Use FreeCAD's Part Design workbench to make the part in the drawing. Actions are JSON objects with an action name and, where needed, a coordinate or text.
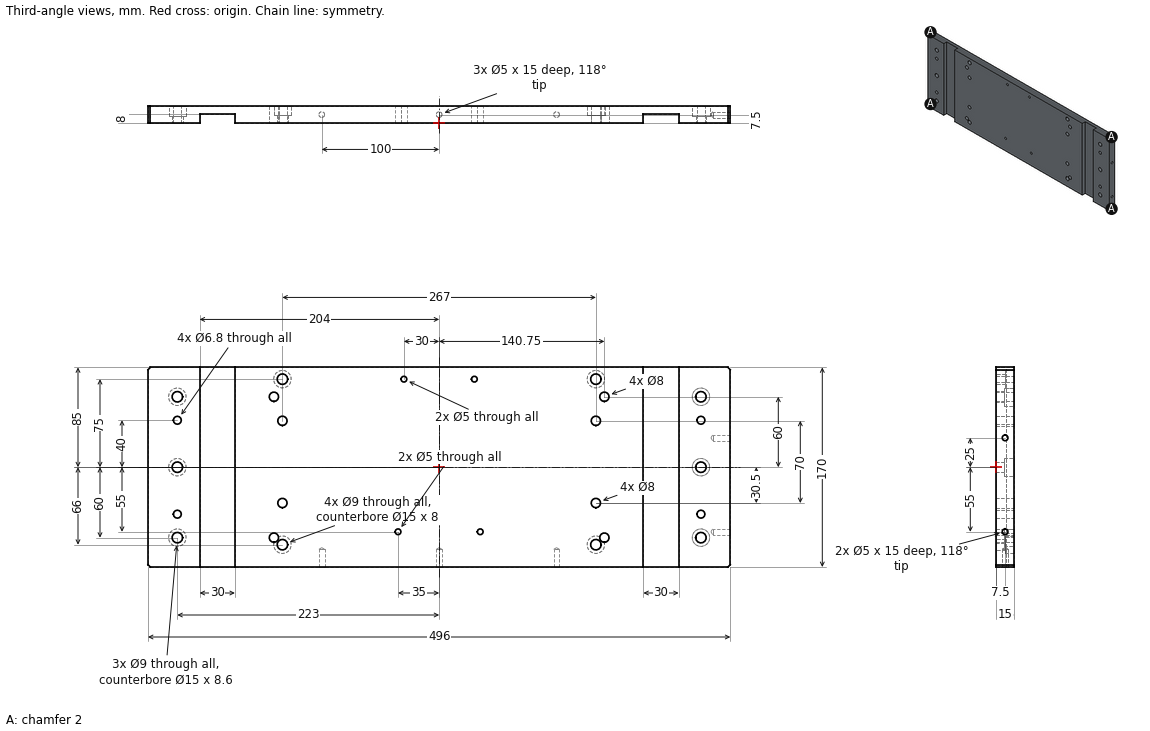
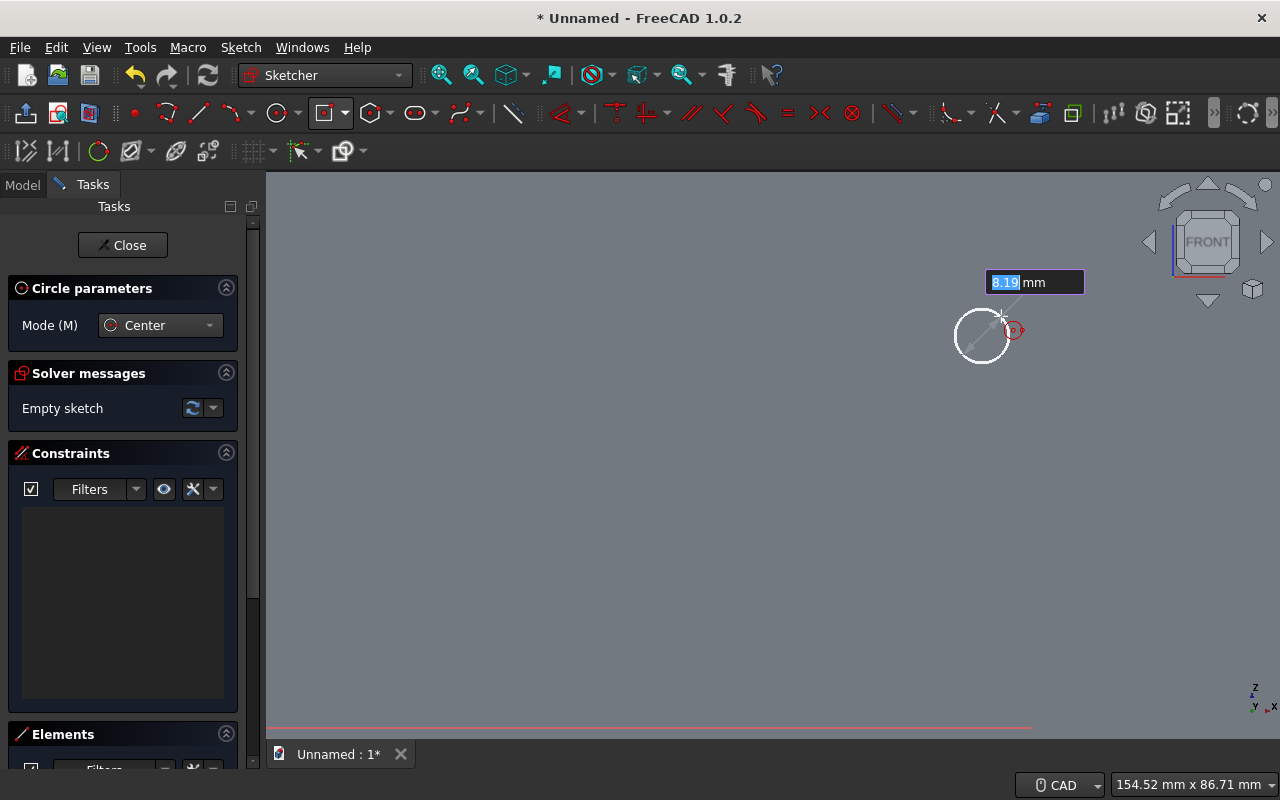
{"action": "type", "text": "8"}
{"action": "key", "text": "Return"}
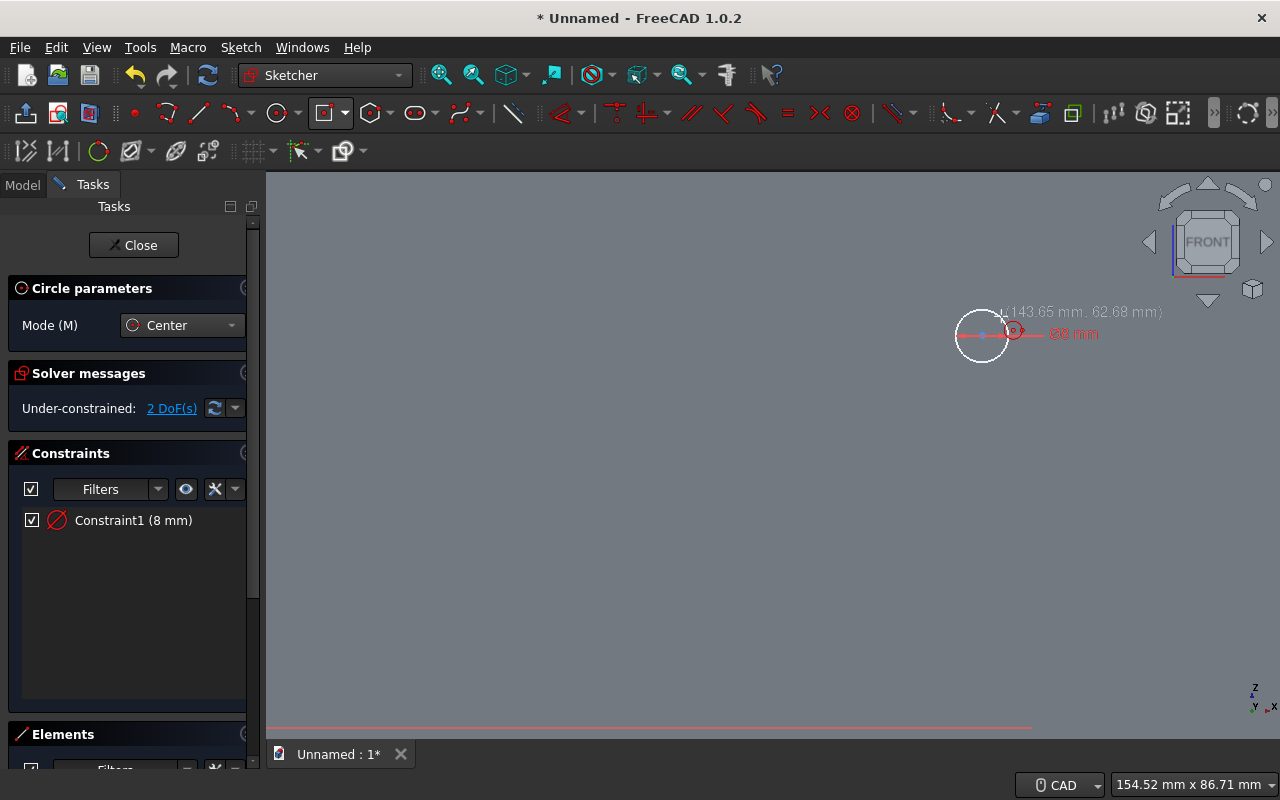
{"action": "scroll", "coordinate": [983, 336], "scroll_direction": "down", "scroll_amount": 6}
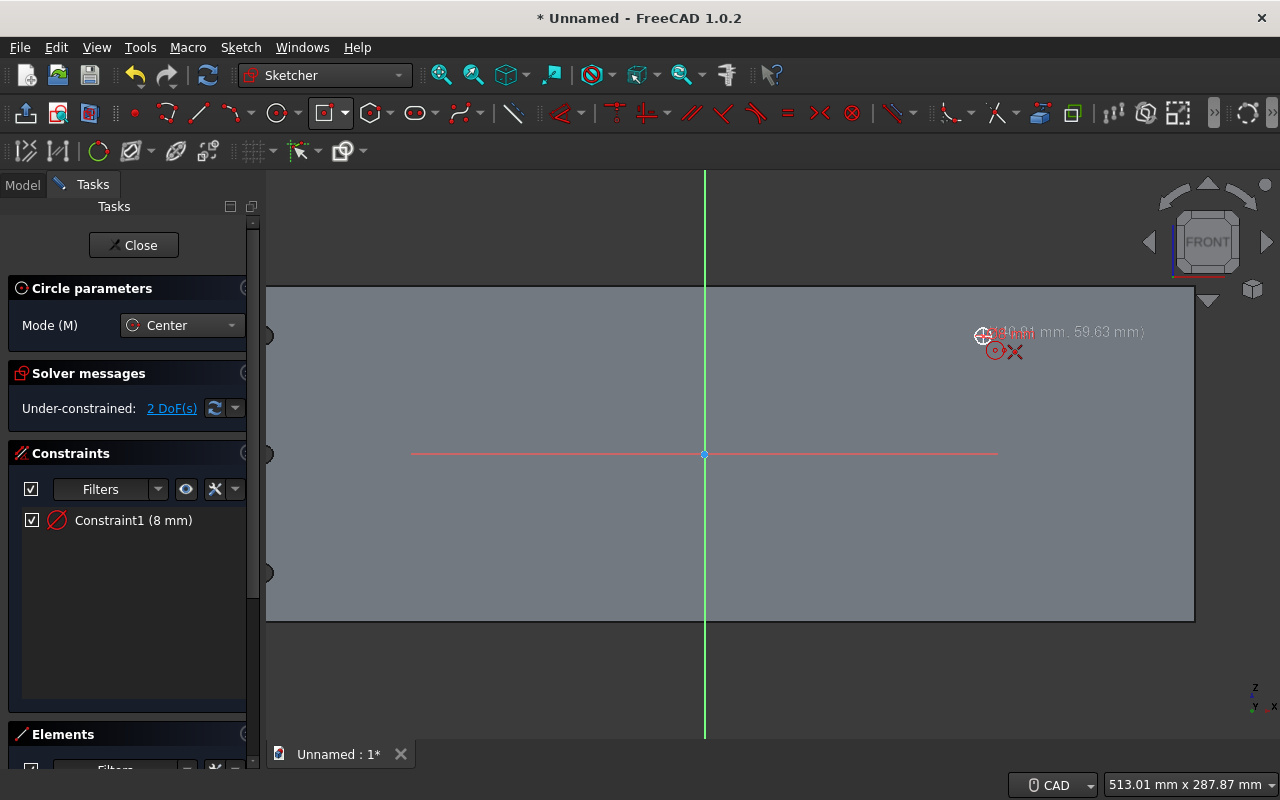
{"action": "scroll", "coordinate": [983, 573], "scroll_direction": "up", "scroll_amount": 6}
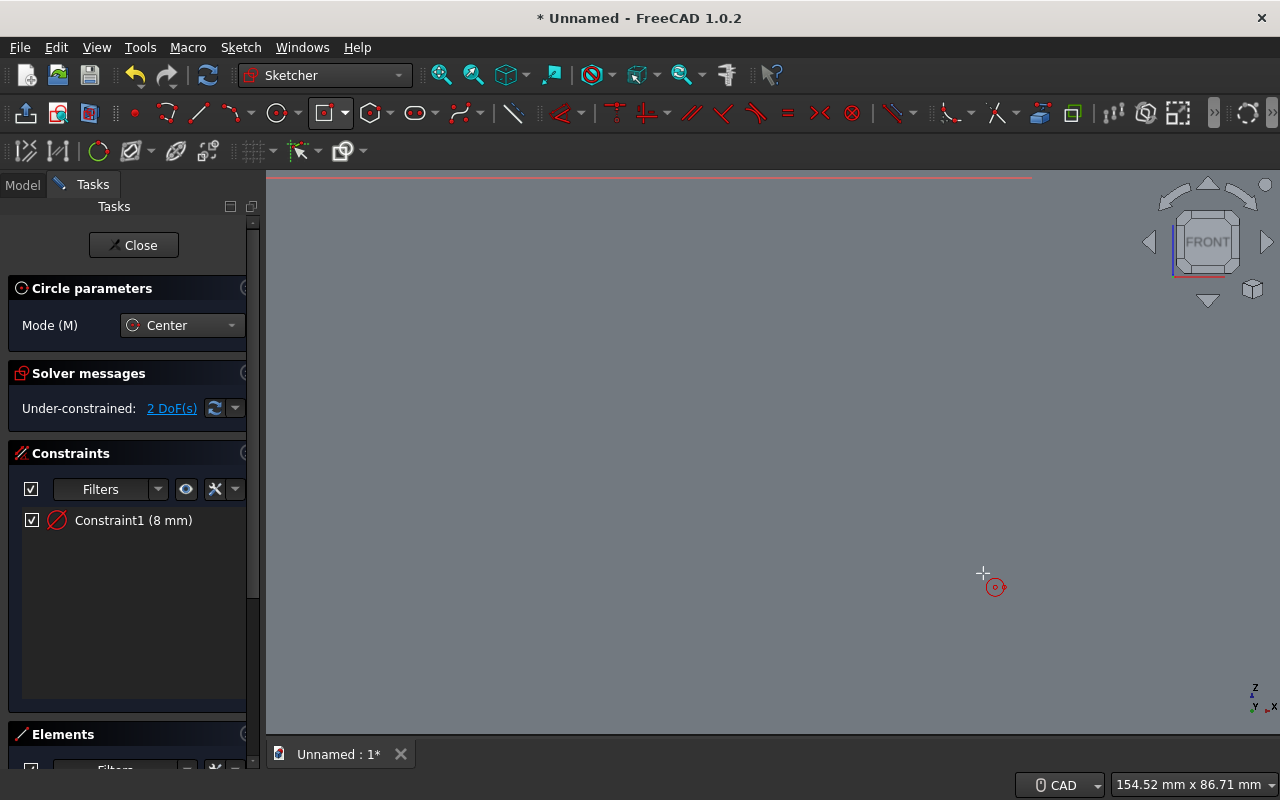
{"action": "left_click", "coordinate": [982, 571]}
{"action": "mouse_move", "coordinate": [1001, 553]}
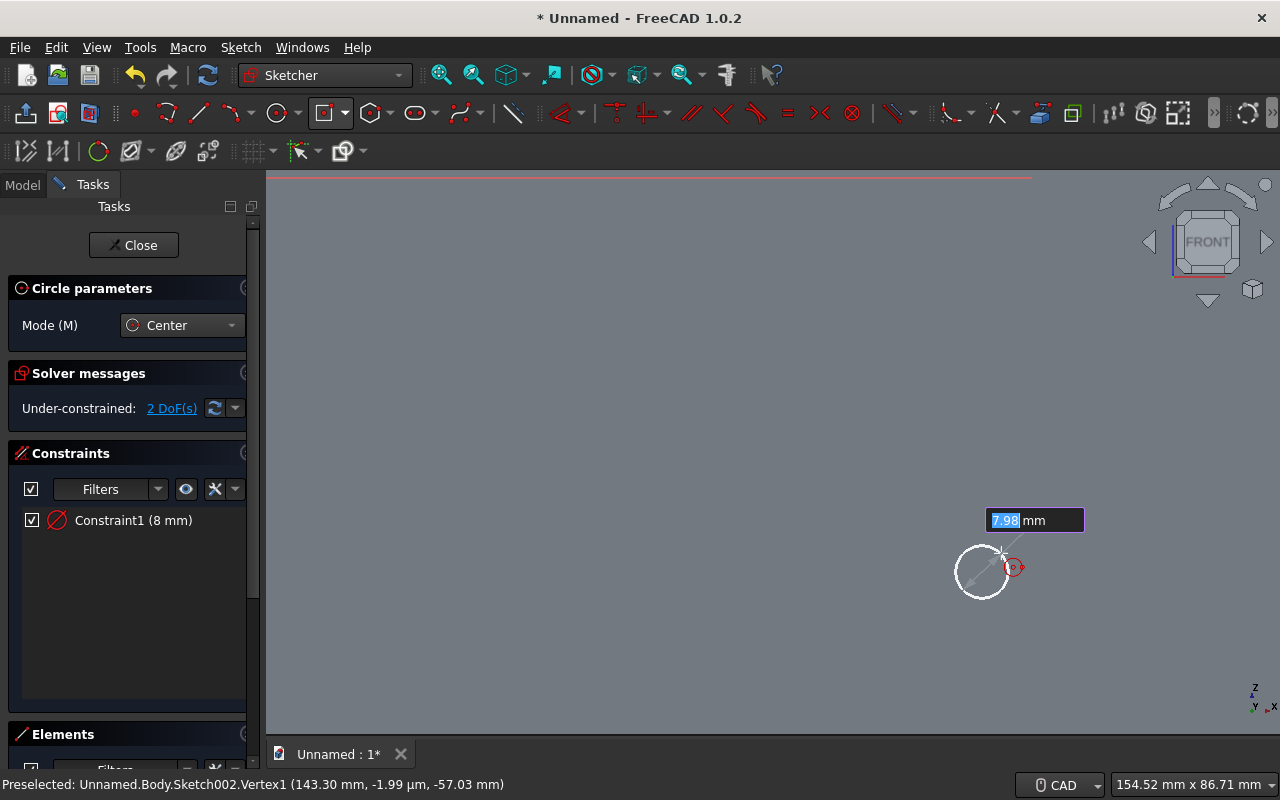
{"action": "type", "text": "8"}
{"action": "key", "text": "Return"}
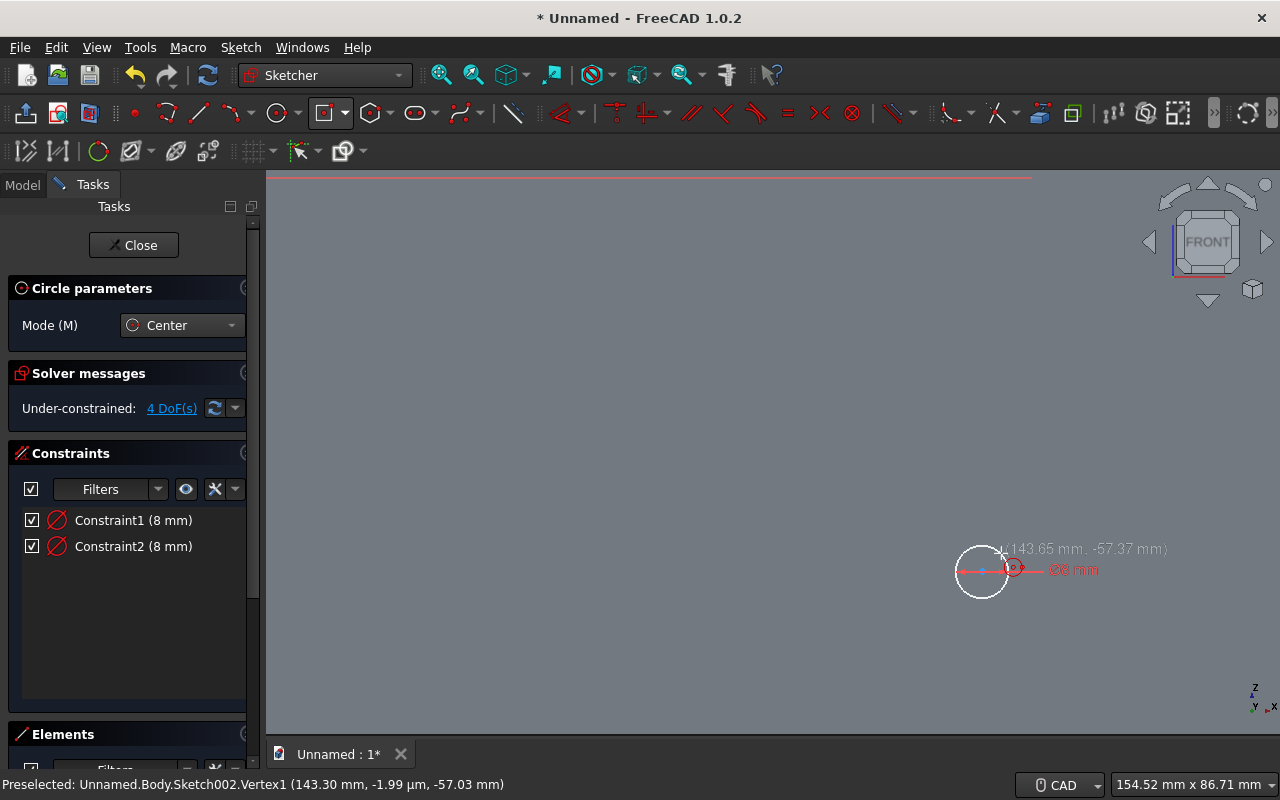
{"action": "scroll", "coordinate": [983, 574], "scroll_direction": "down", "scroll_amount": 6}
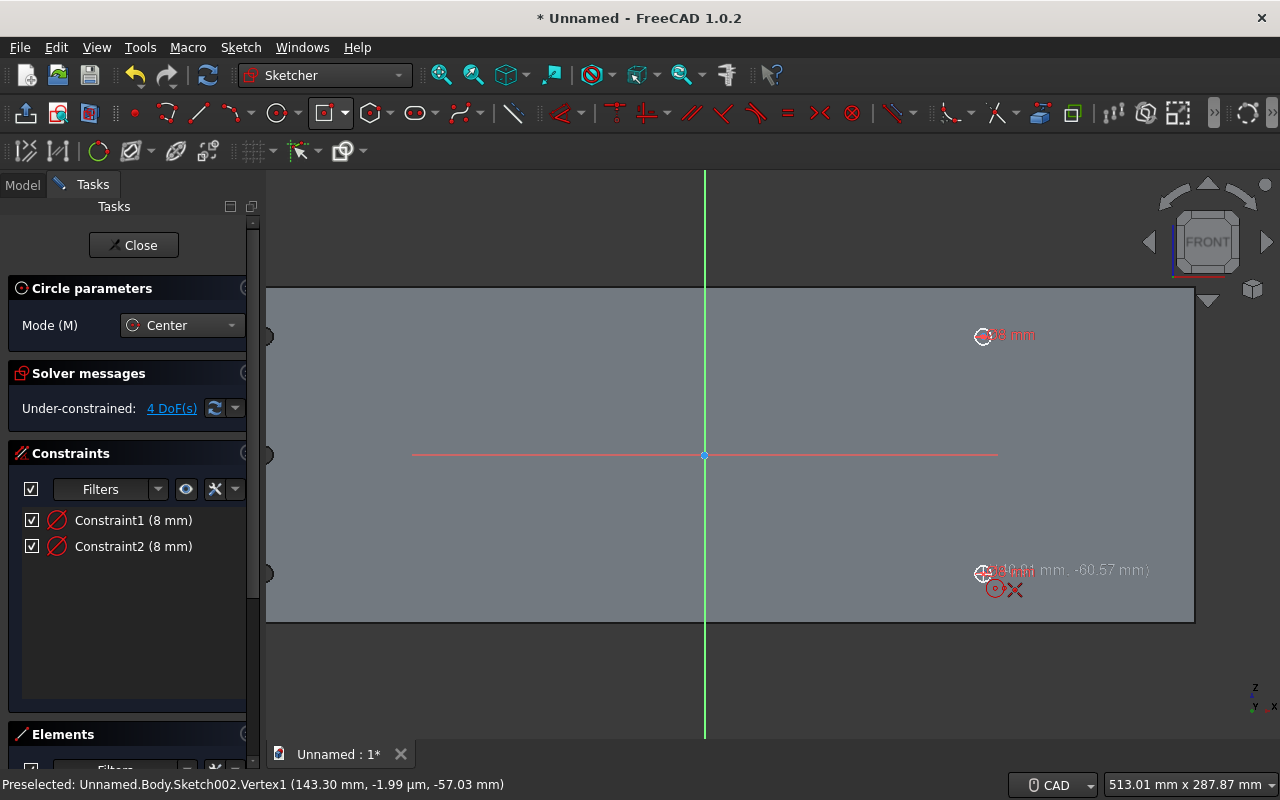
{"action": "scroll", "coordinate": [427, 574], "scroll_direction": "up", "scroll_amount": 6}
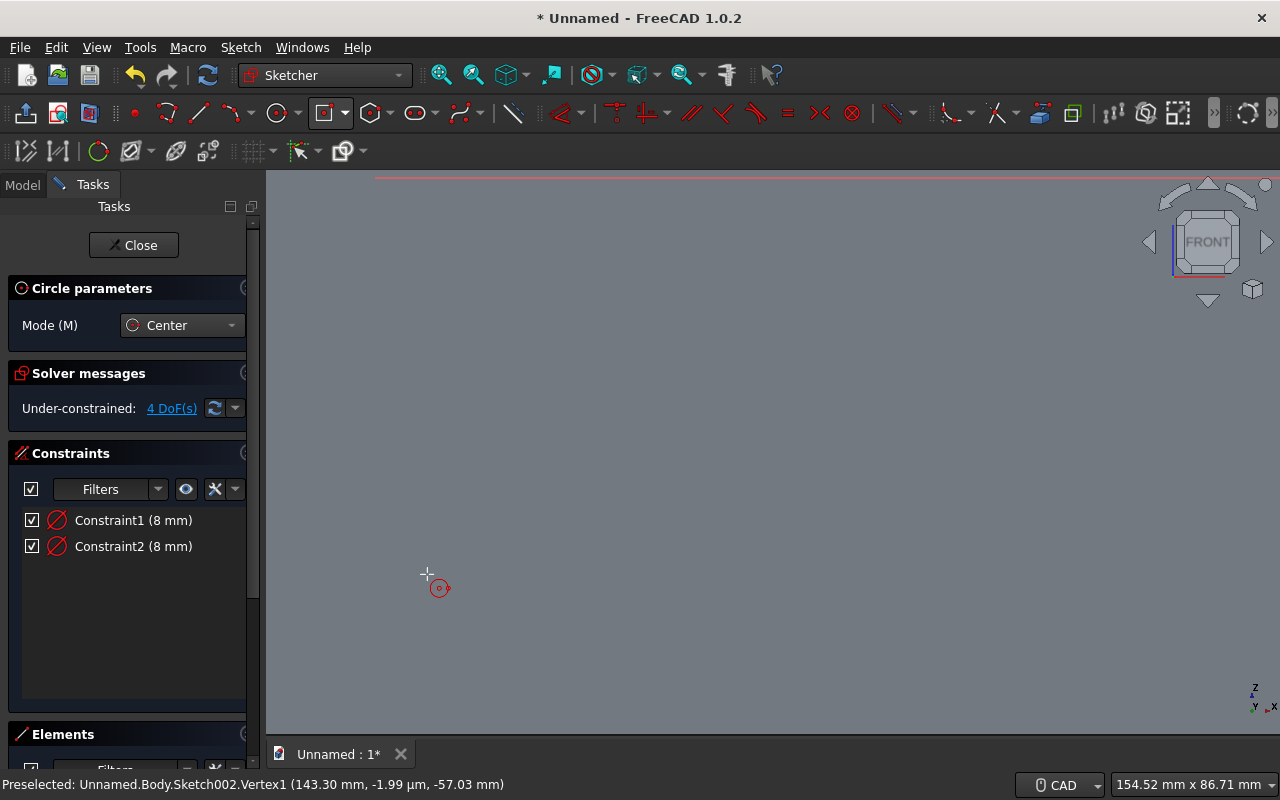
{"action": "left_click", "coordinate": [426, 571]}
{"action": "mouse_move", "coordinate": [444, 553]}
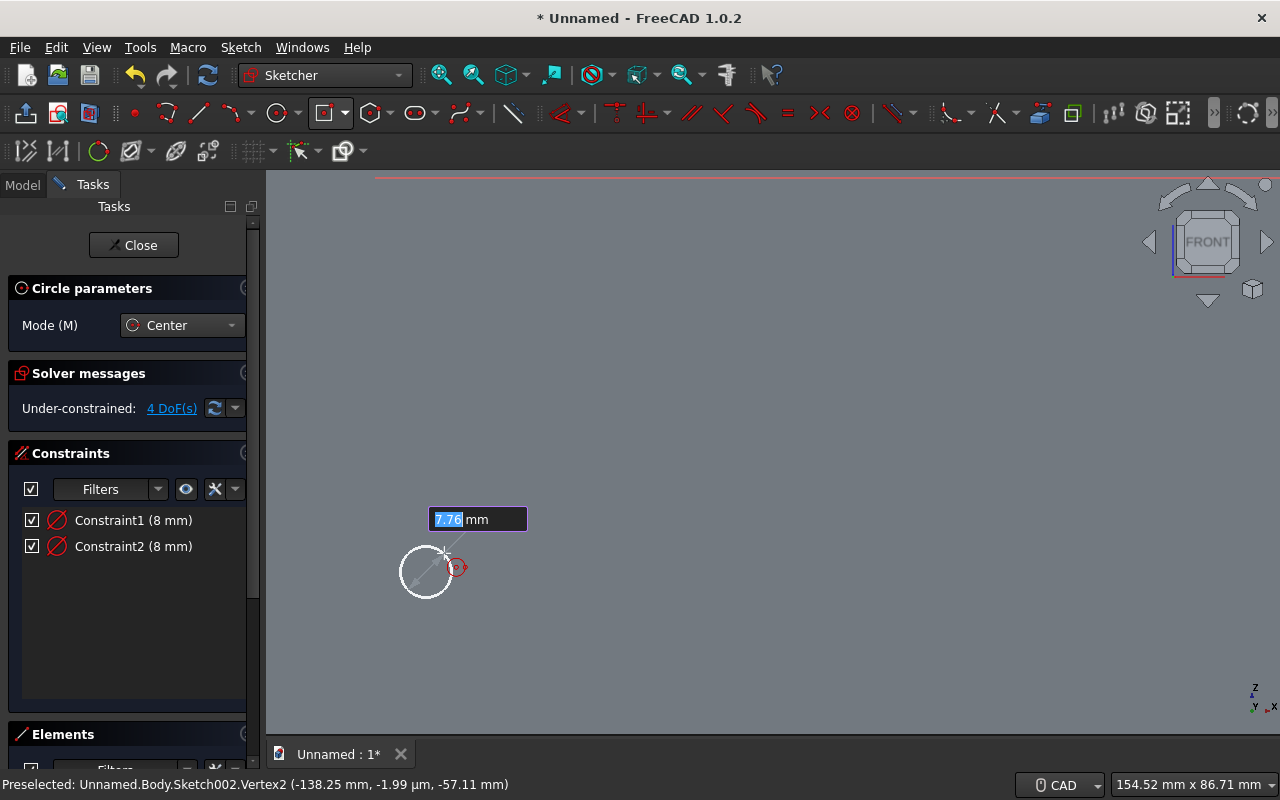
{"action": "type", "text": "8"}
{"action": "key", "text": "Return"}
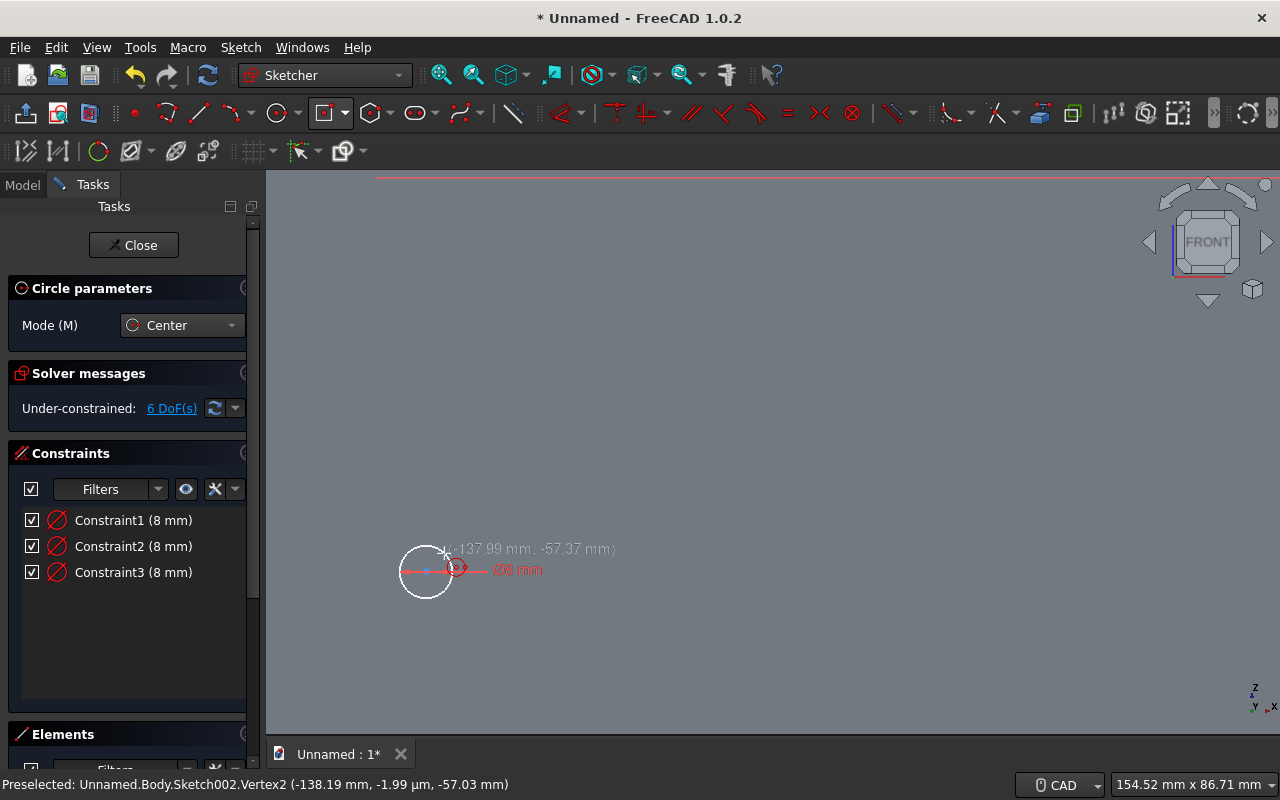
{"action": "scroll", "coordinate": [426, 574], "scroll_direction": "down", "scroll_amount": 6}